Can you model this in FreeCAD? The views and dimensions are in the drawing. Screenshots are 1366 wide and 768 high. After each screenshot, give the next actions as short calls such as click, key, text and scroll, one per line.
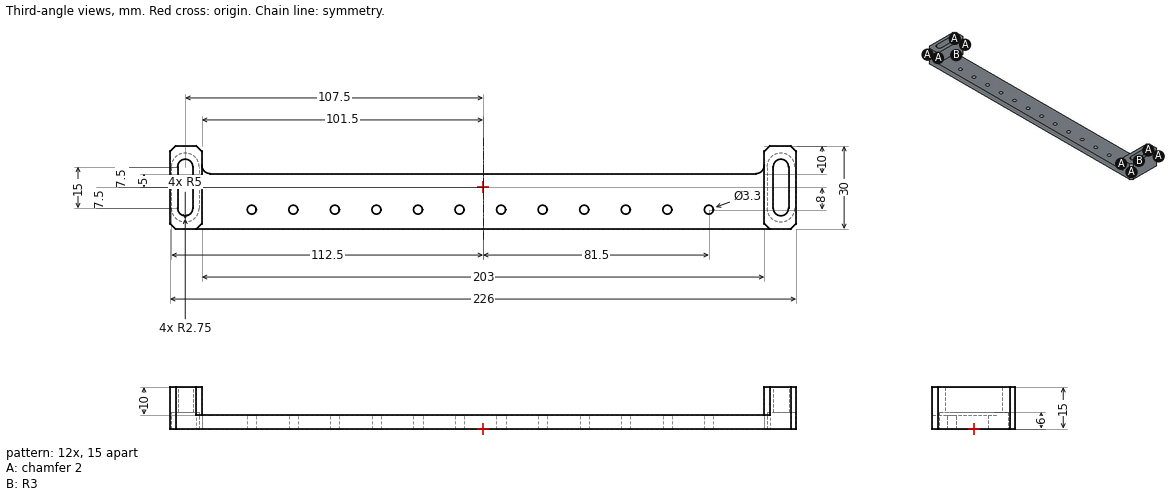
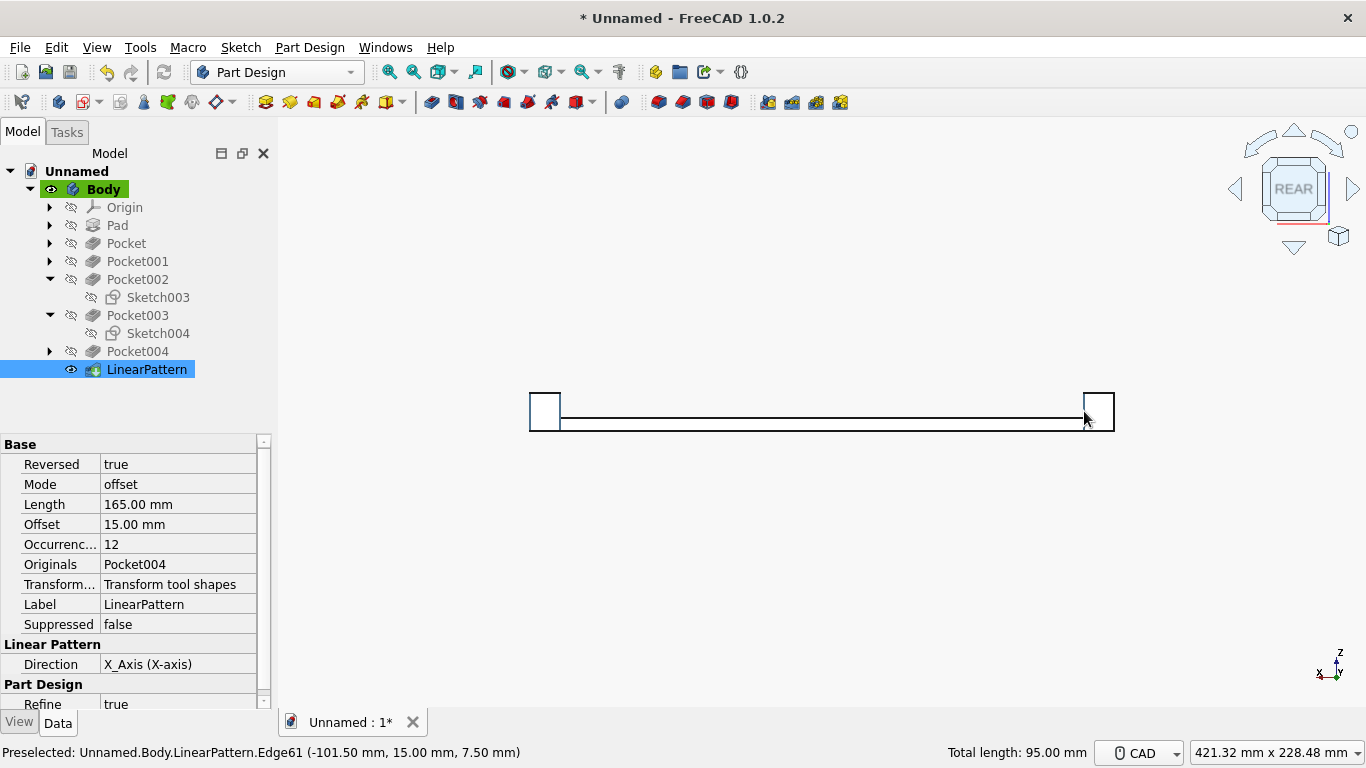
click(1114, 411, ctrl)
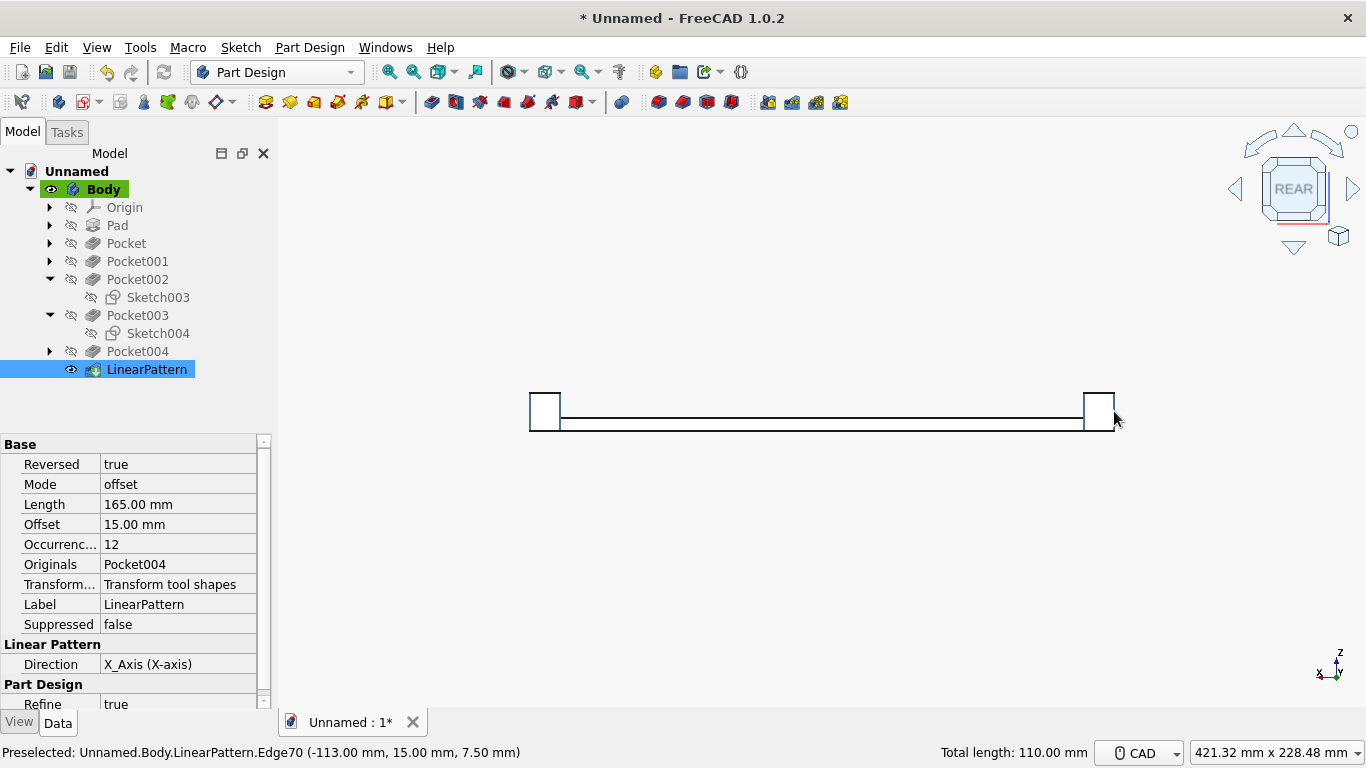
click(684, 102)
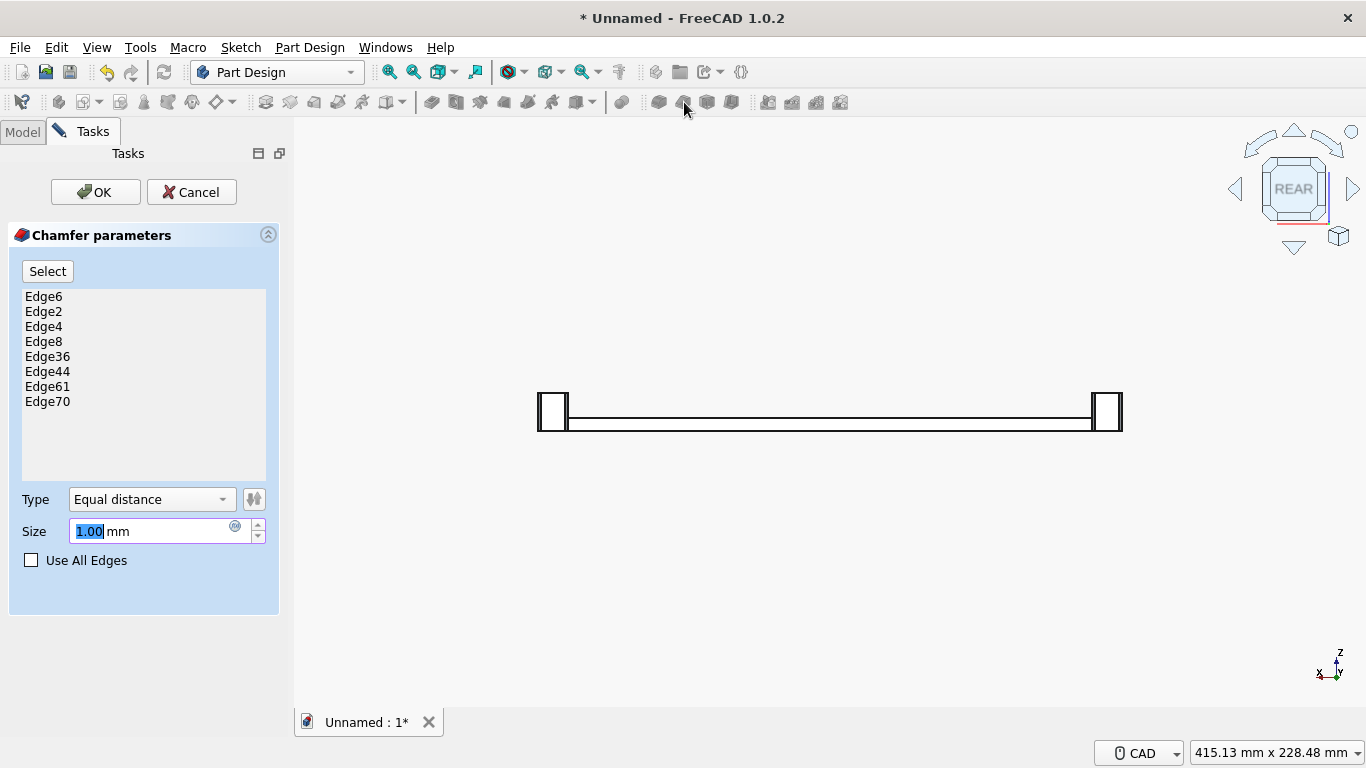
text(2)
key(Tab)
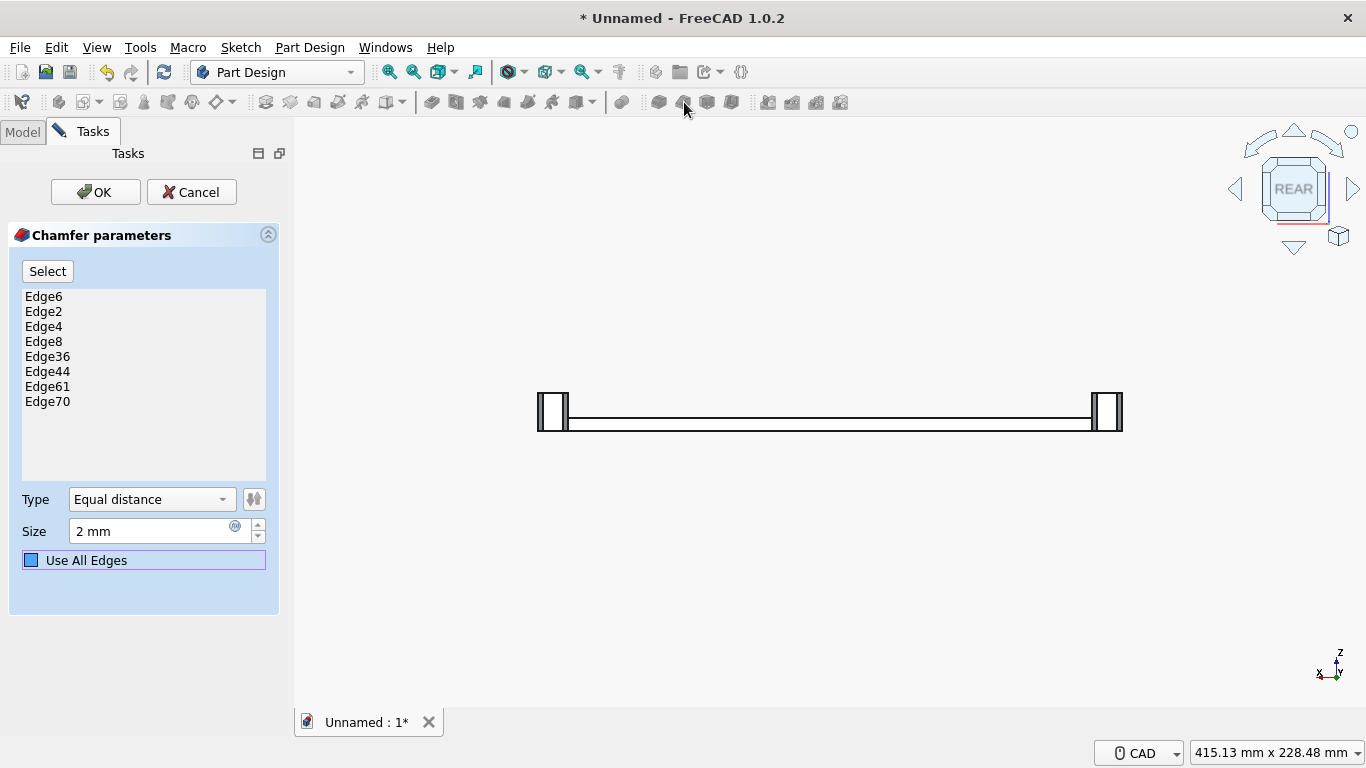
click(96, 192)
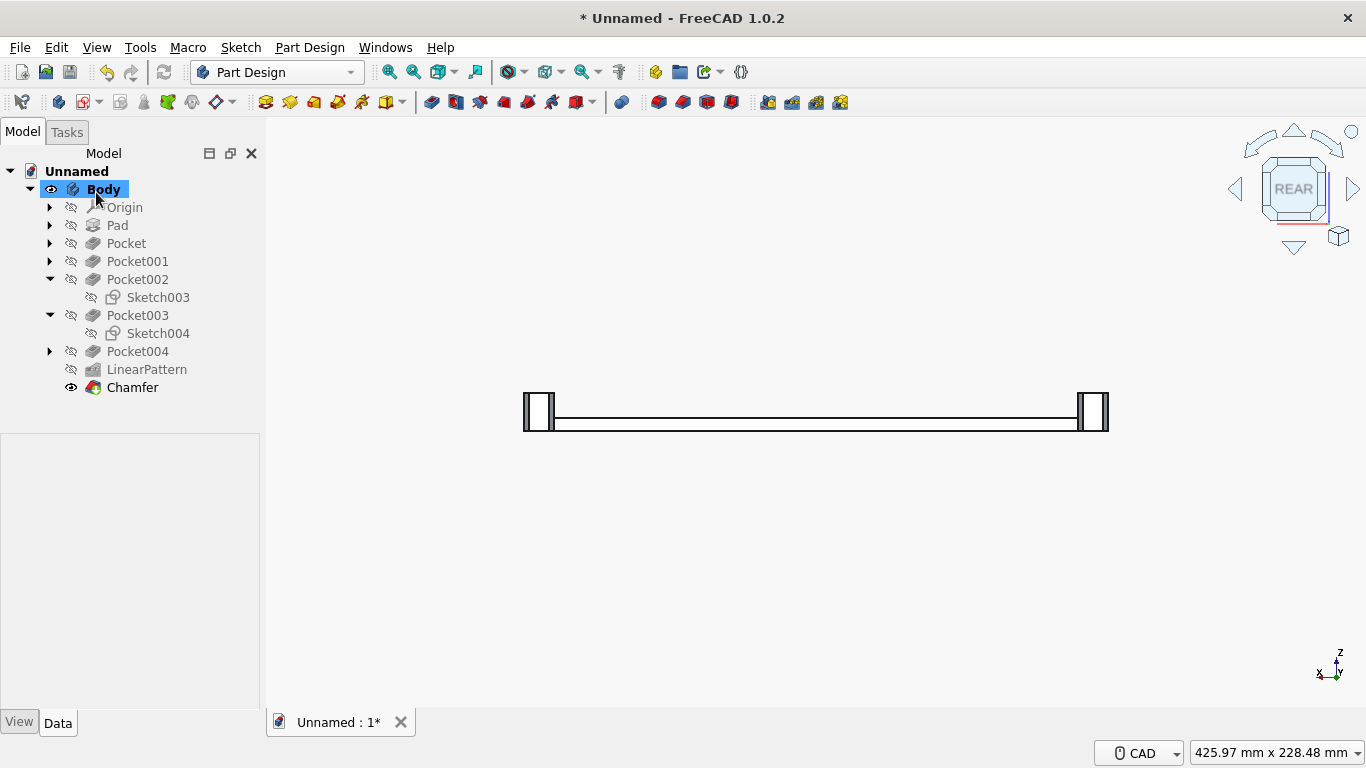
scroll(1078, 424, up, 6)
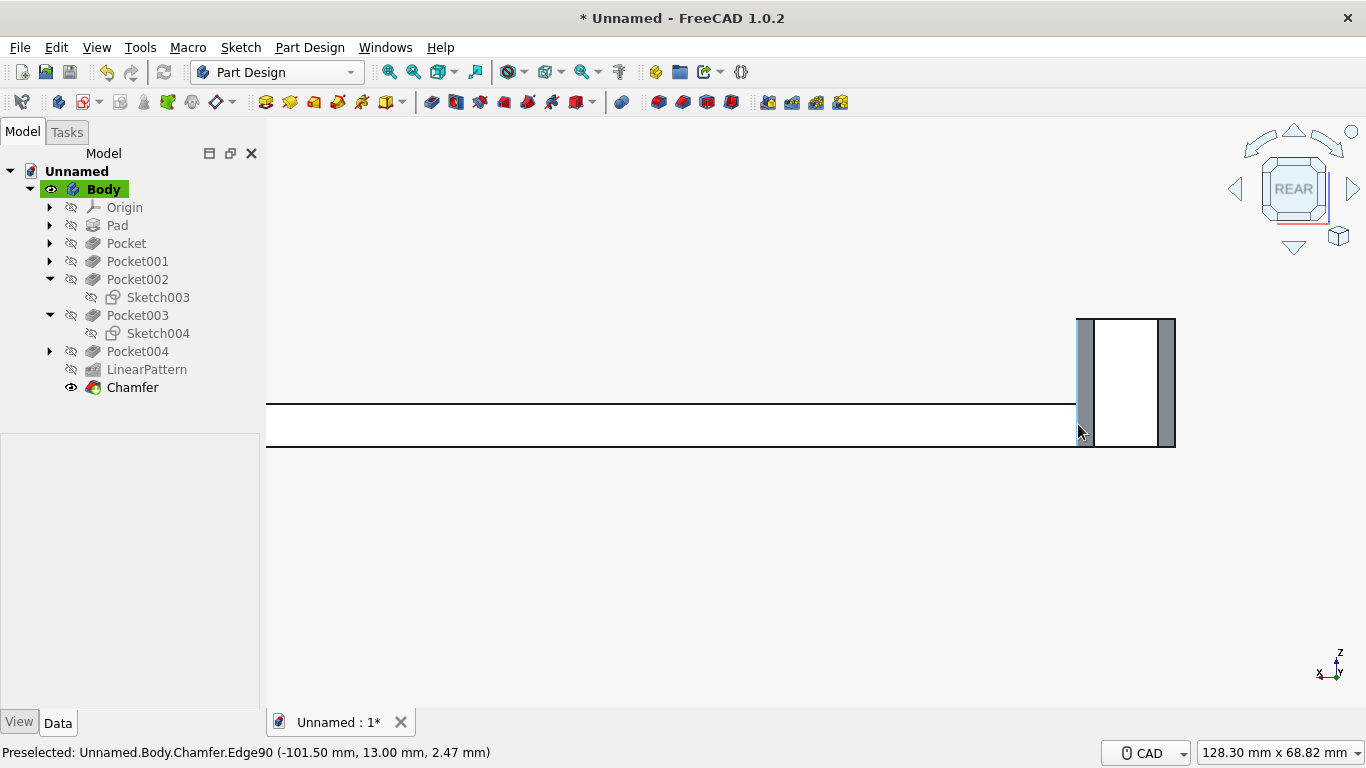
key(v)
key(f)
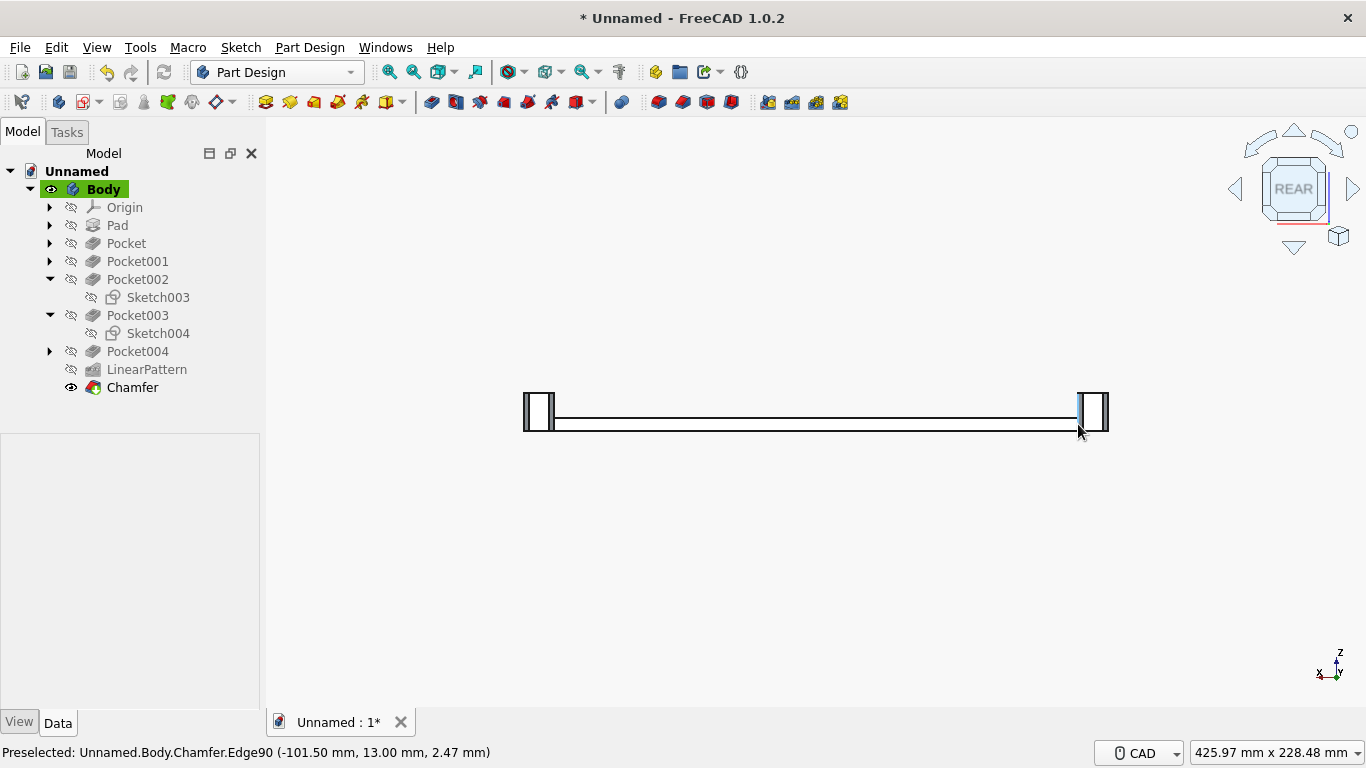
key(0)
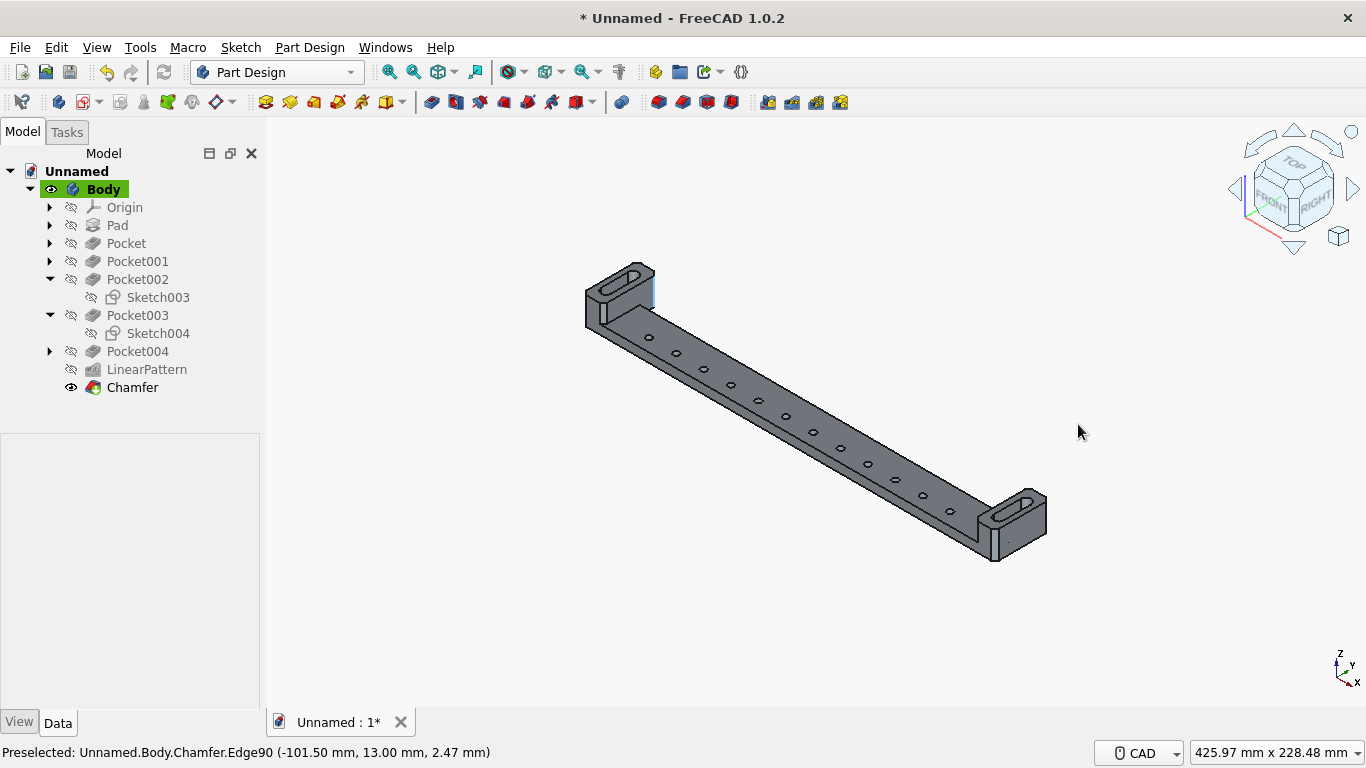
scroll(640, 309, up, 6)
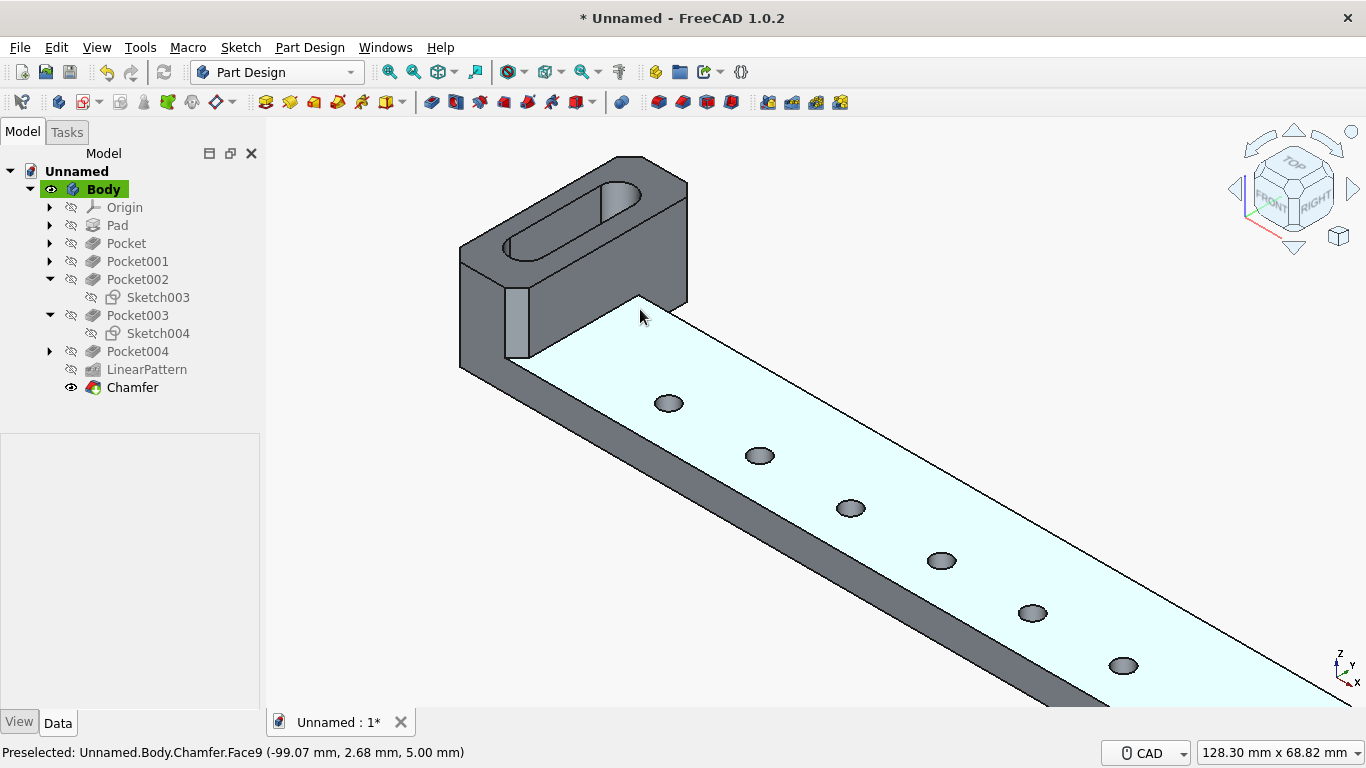
key(v)
key(f)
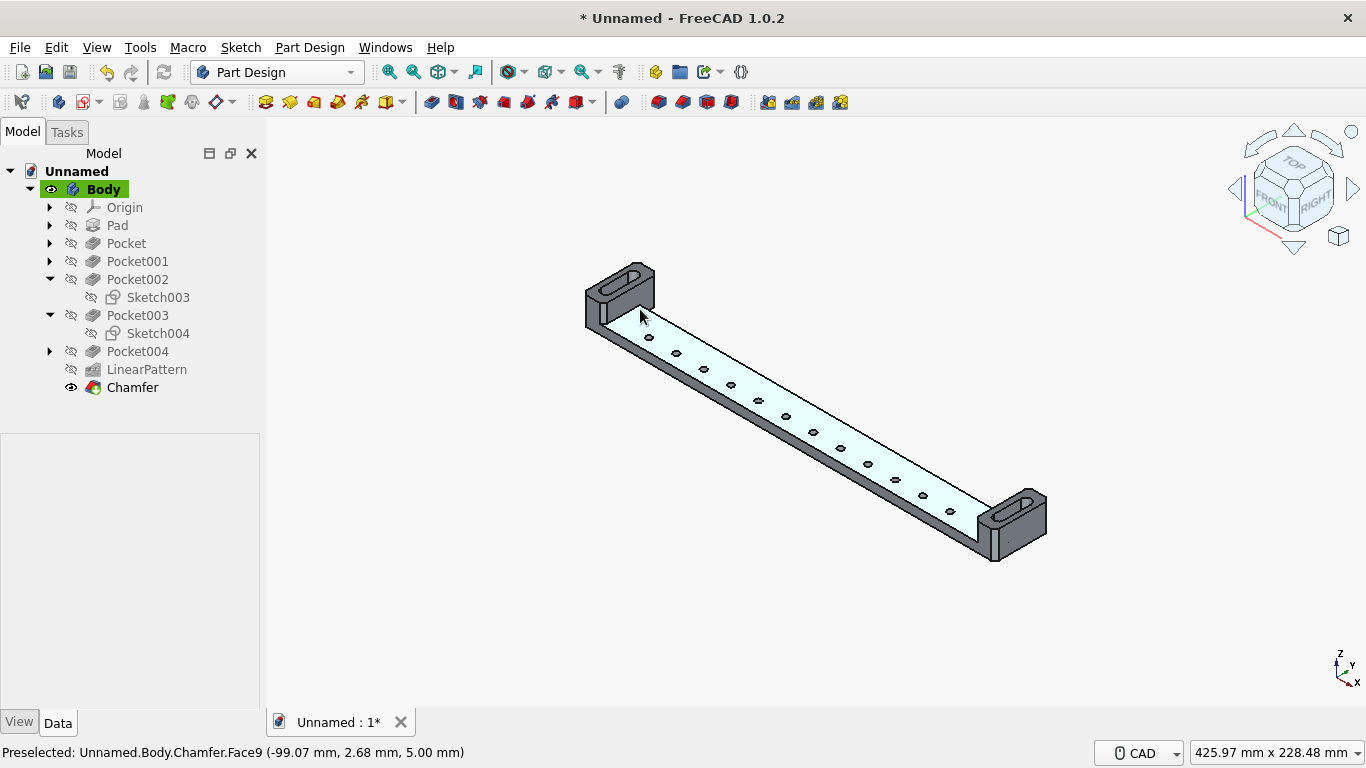
key(2)